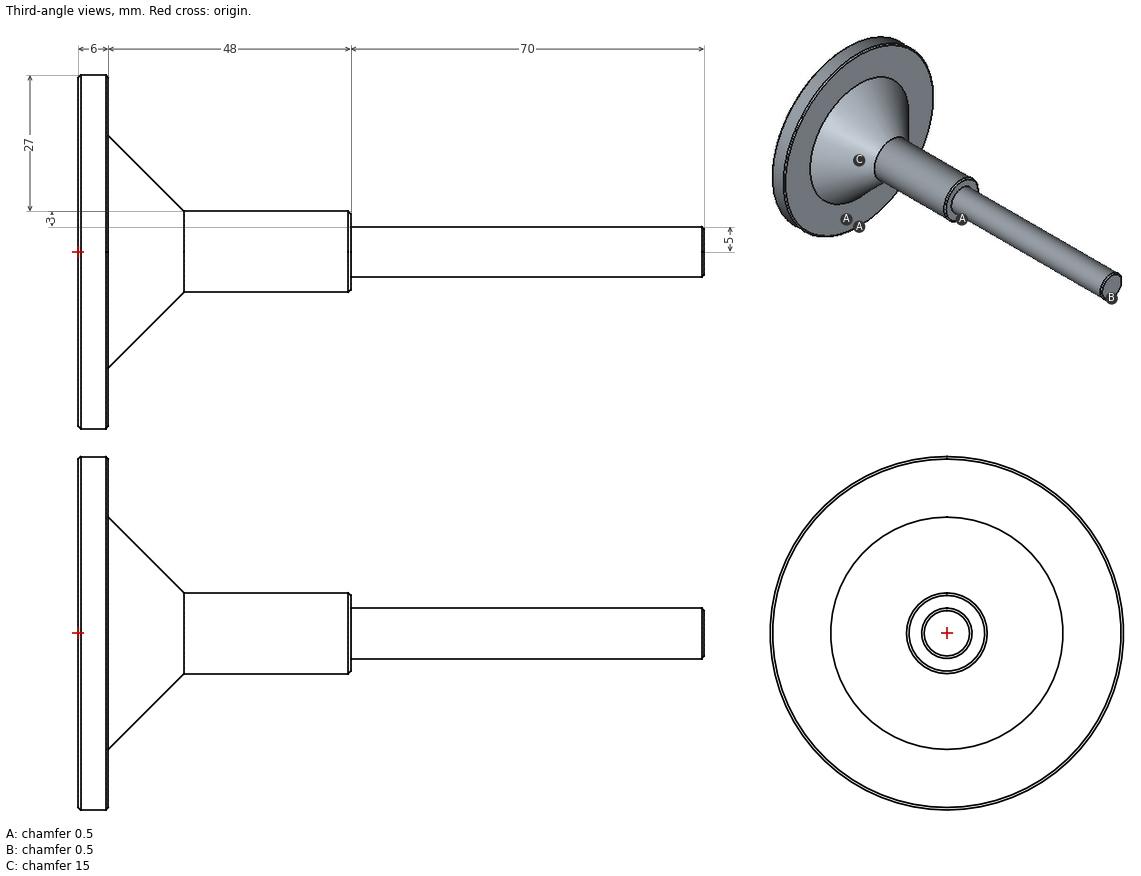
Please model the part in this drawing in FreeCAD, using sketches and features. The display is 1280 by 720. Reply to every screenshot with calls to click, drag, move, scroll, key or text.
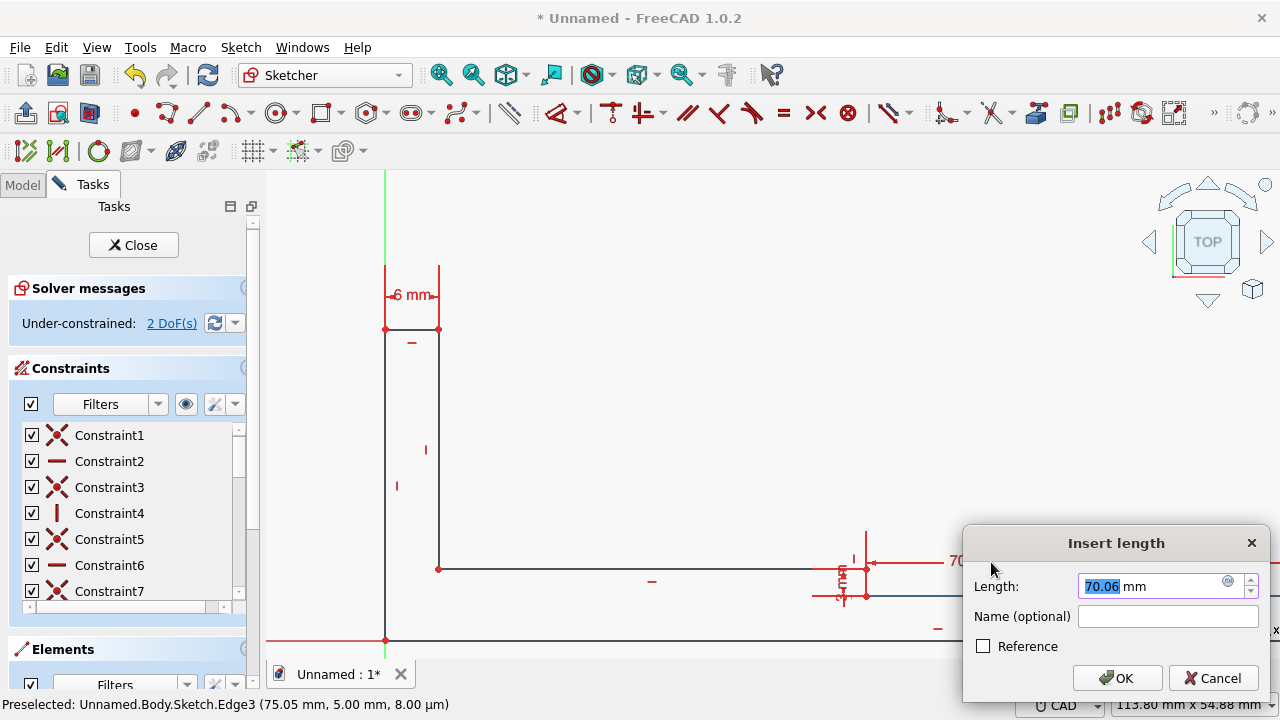
text(70)
key(Return)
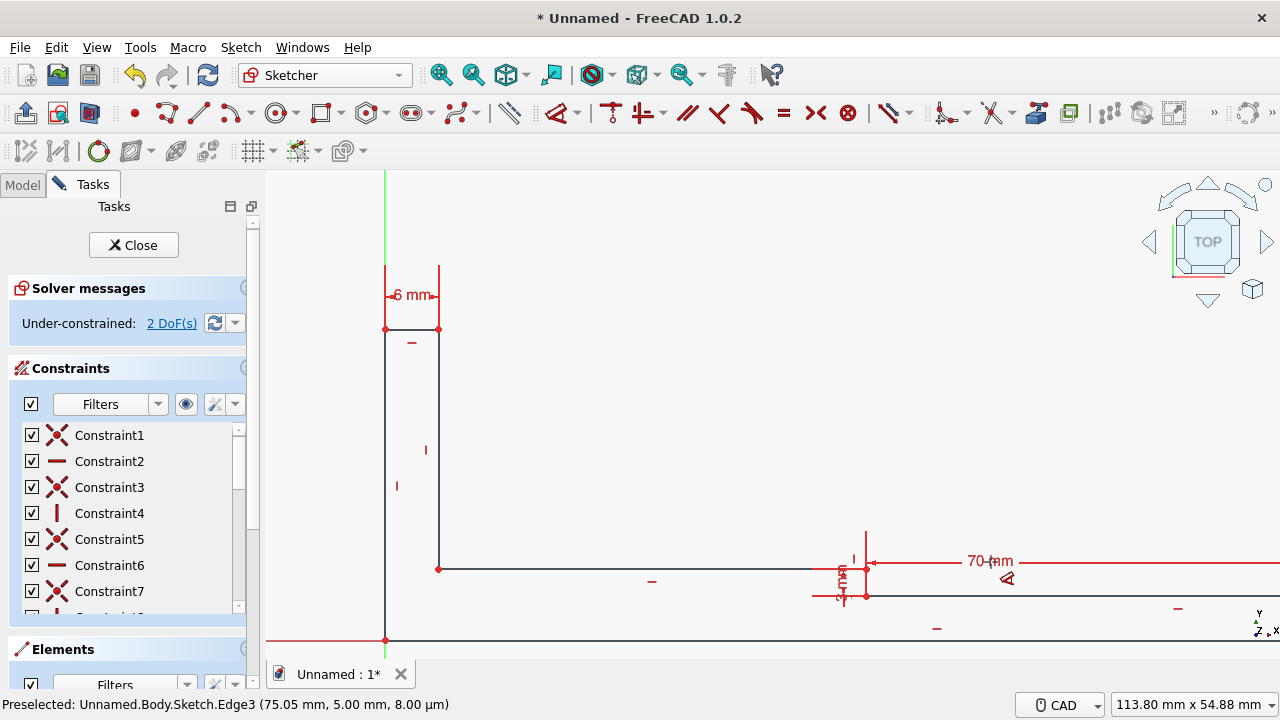
click(738, 569)
click(653, 603)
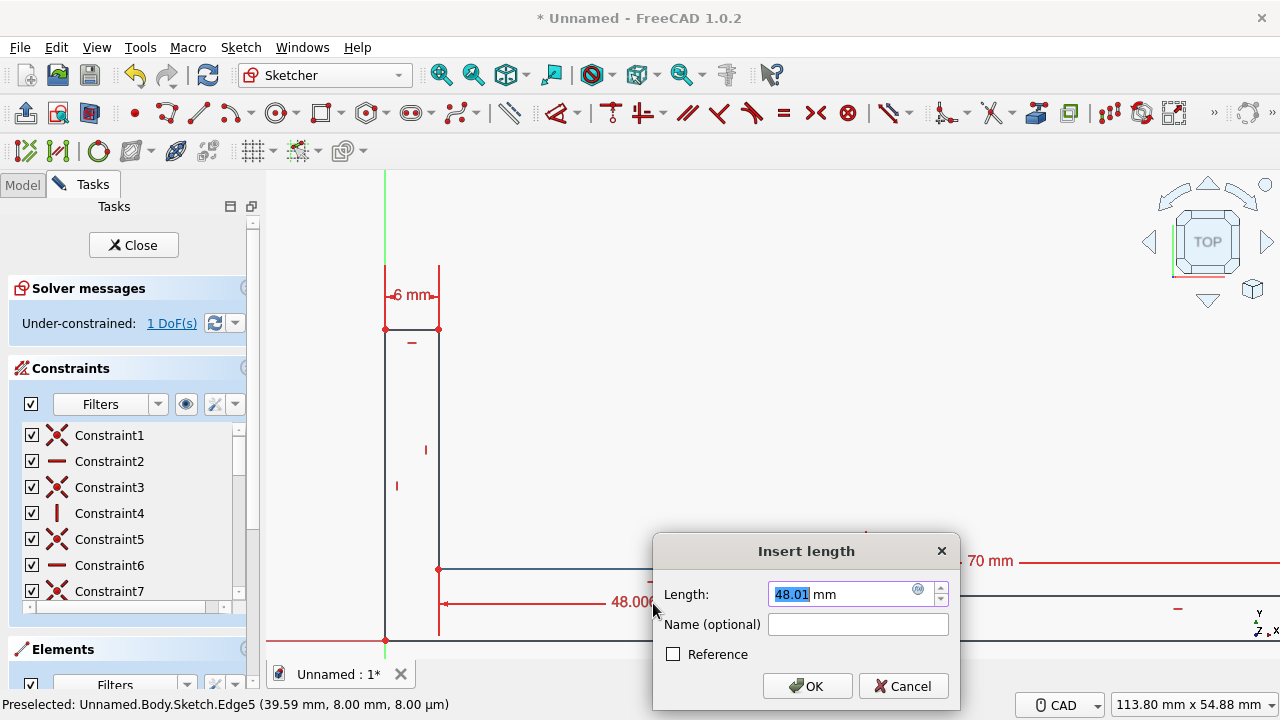
text(48)
key(Return)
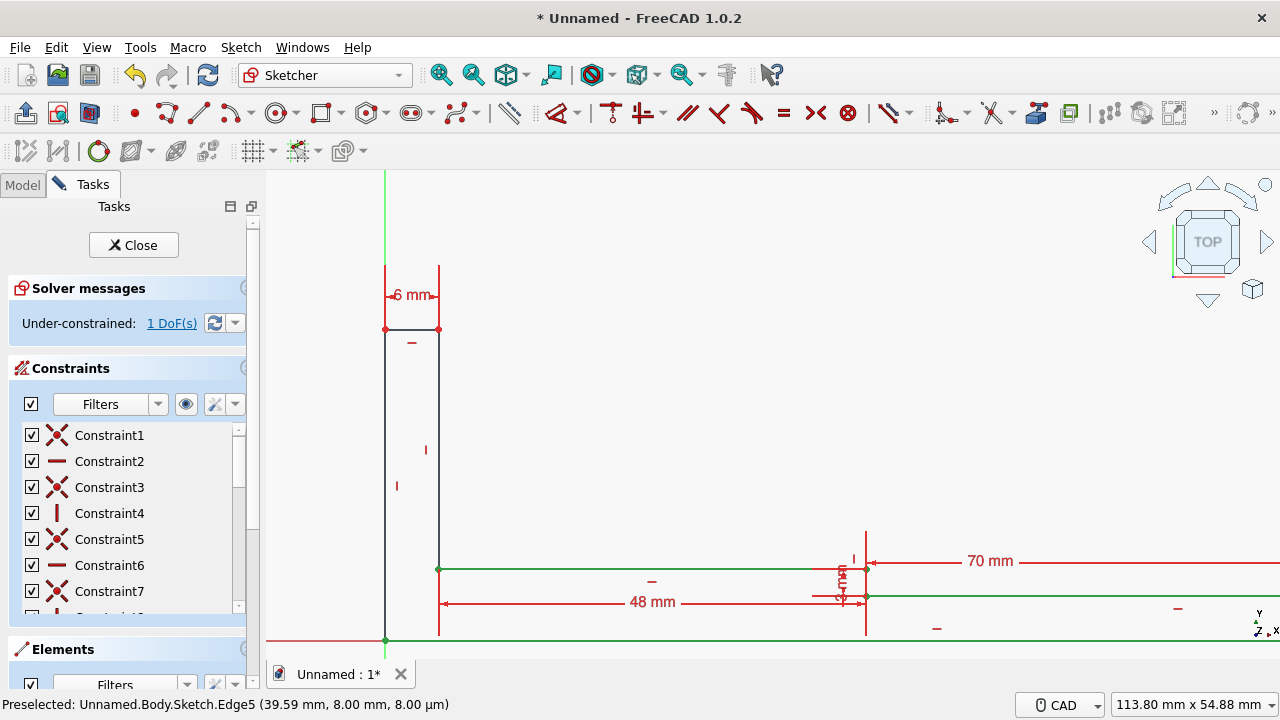
click(439, 498)
click(405, 450)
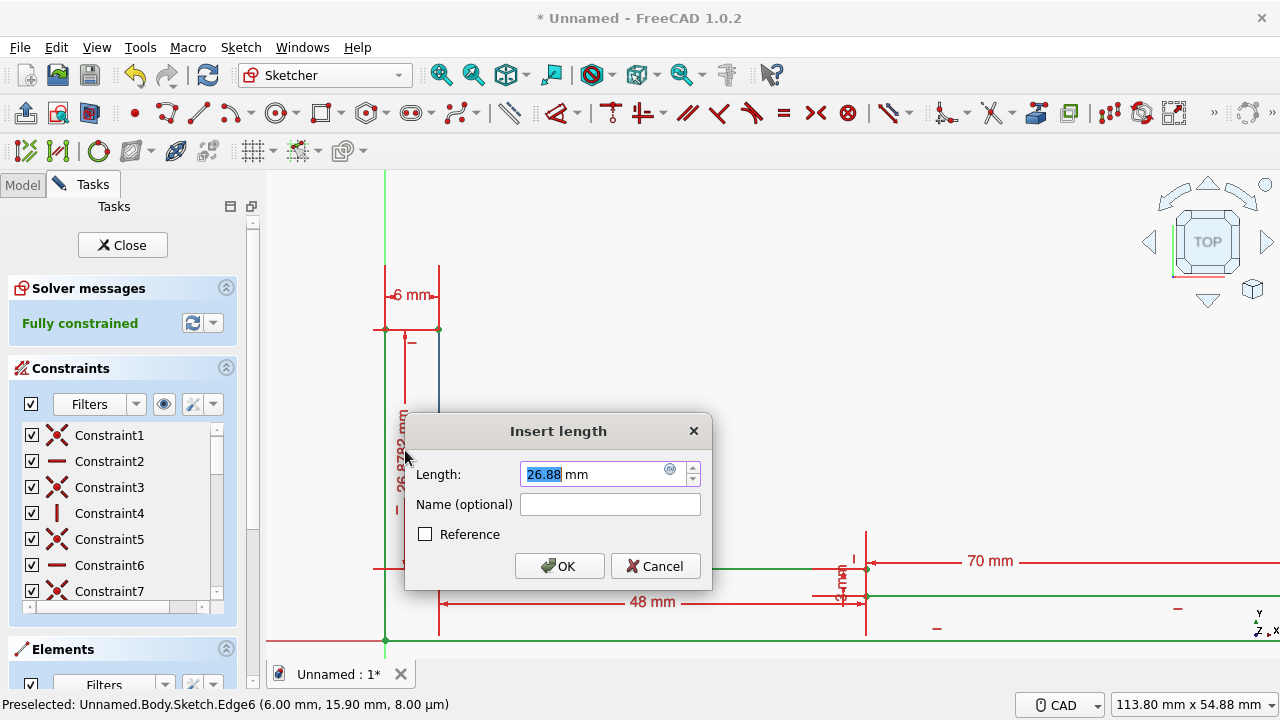
text(27)
key(Return)
key(Escape)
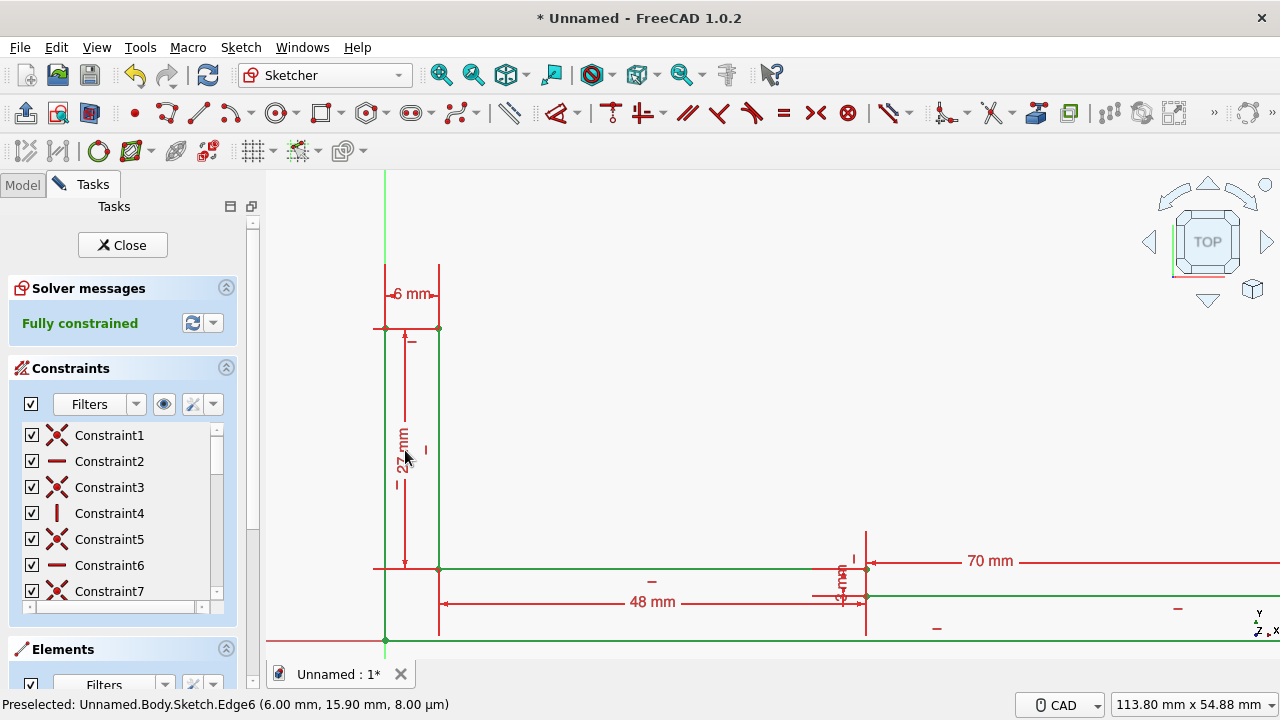
click(123, 245)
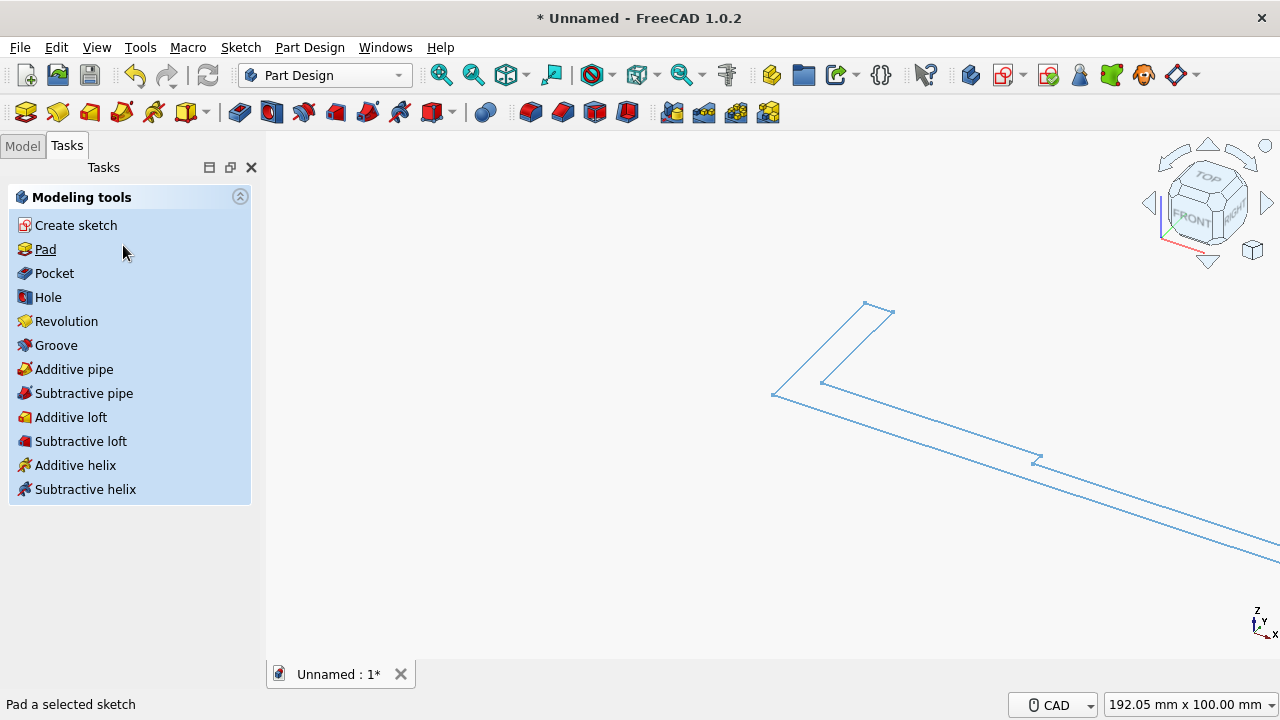
click(58, 112)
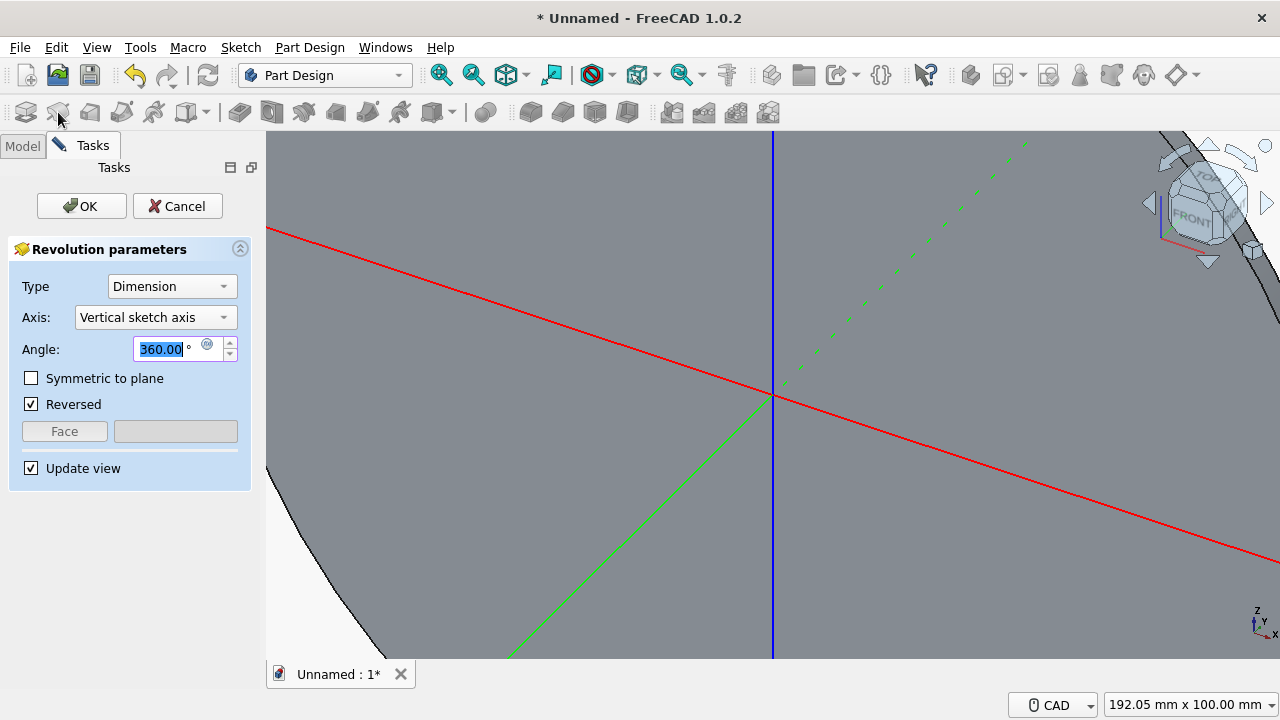
click(156, 318)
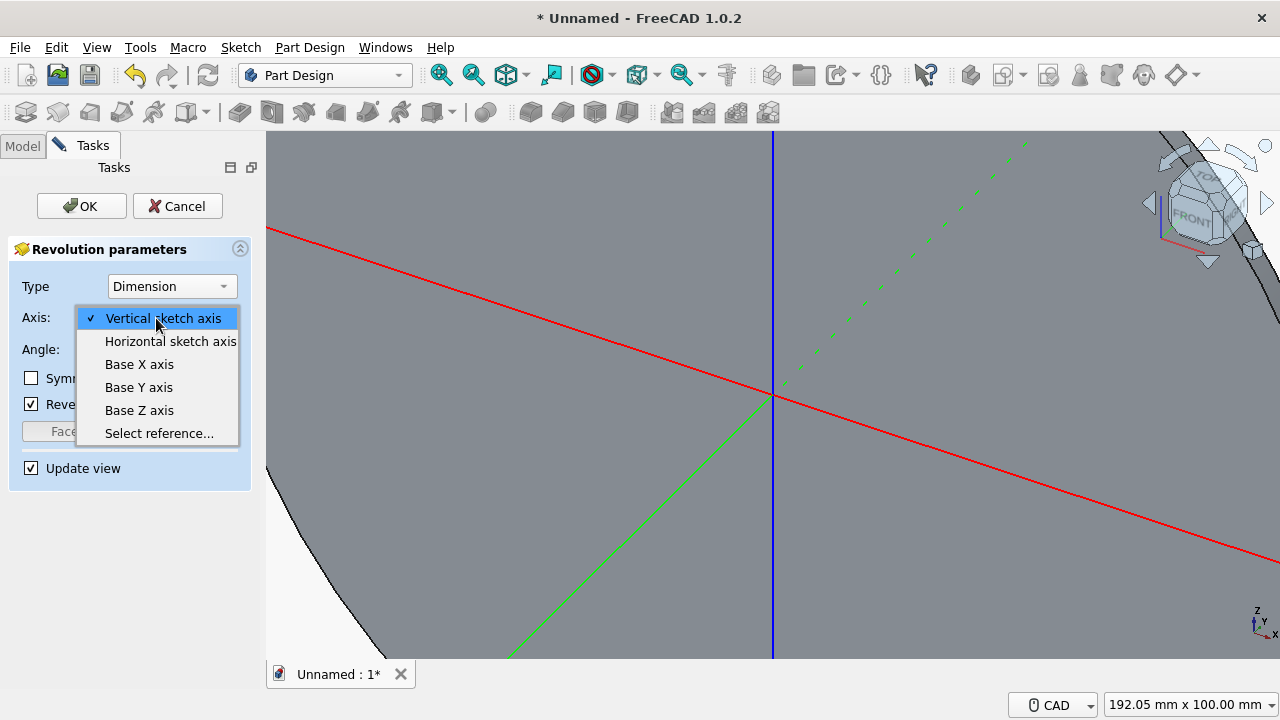
click(156, 342)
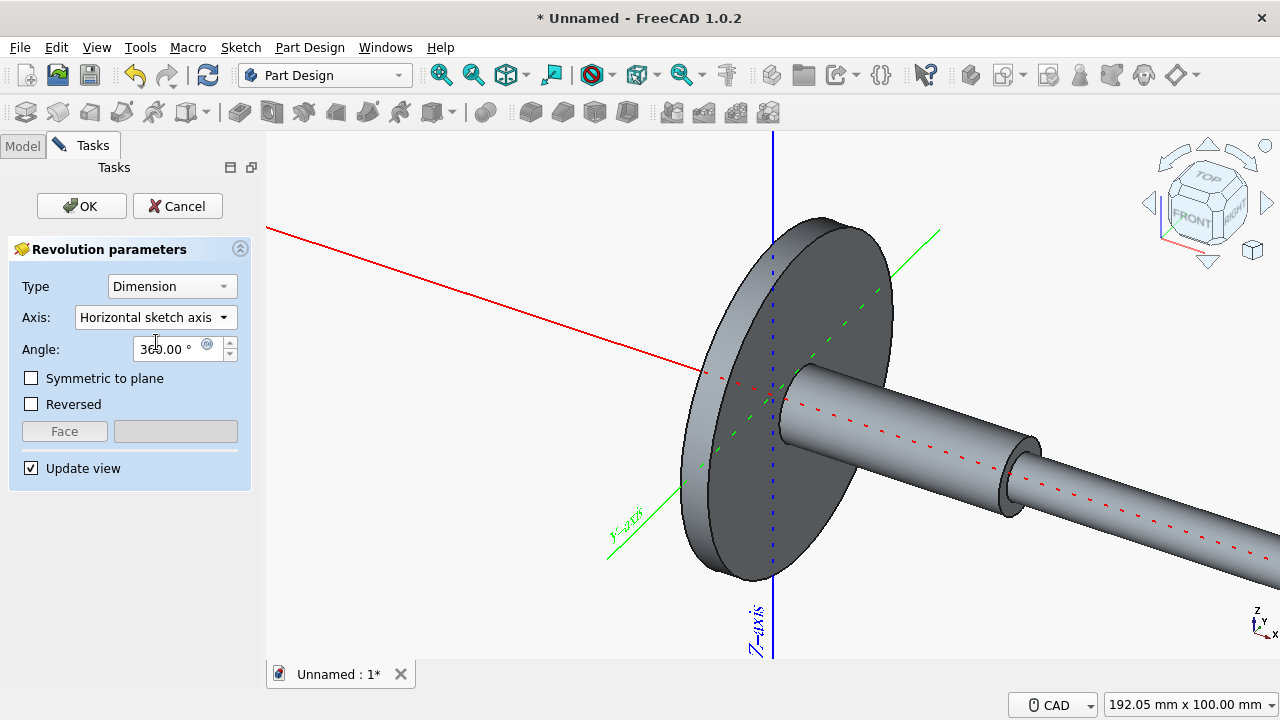
click(82, 206)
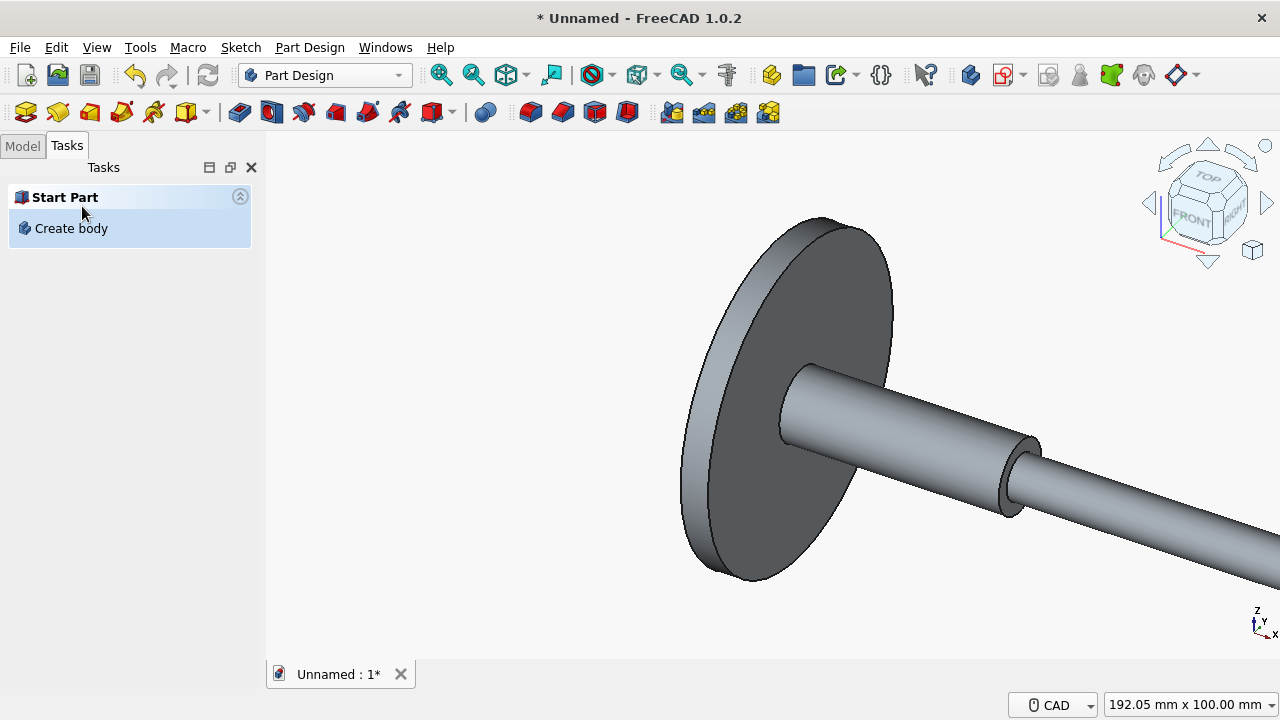
click(442, 76)